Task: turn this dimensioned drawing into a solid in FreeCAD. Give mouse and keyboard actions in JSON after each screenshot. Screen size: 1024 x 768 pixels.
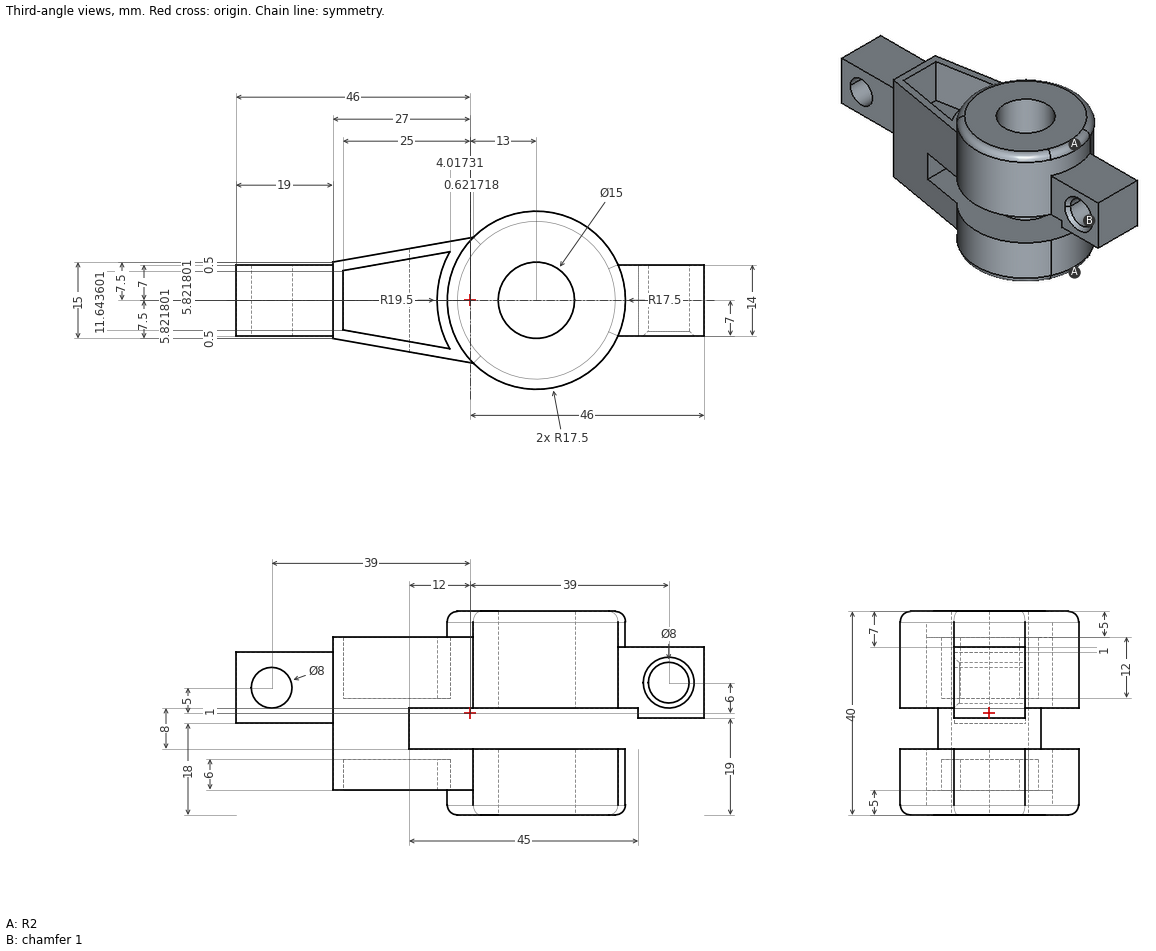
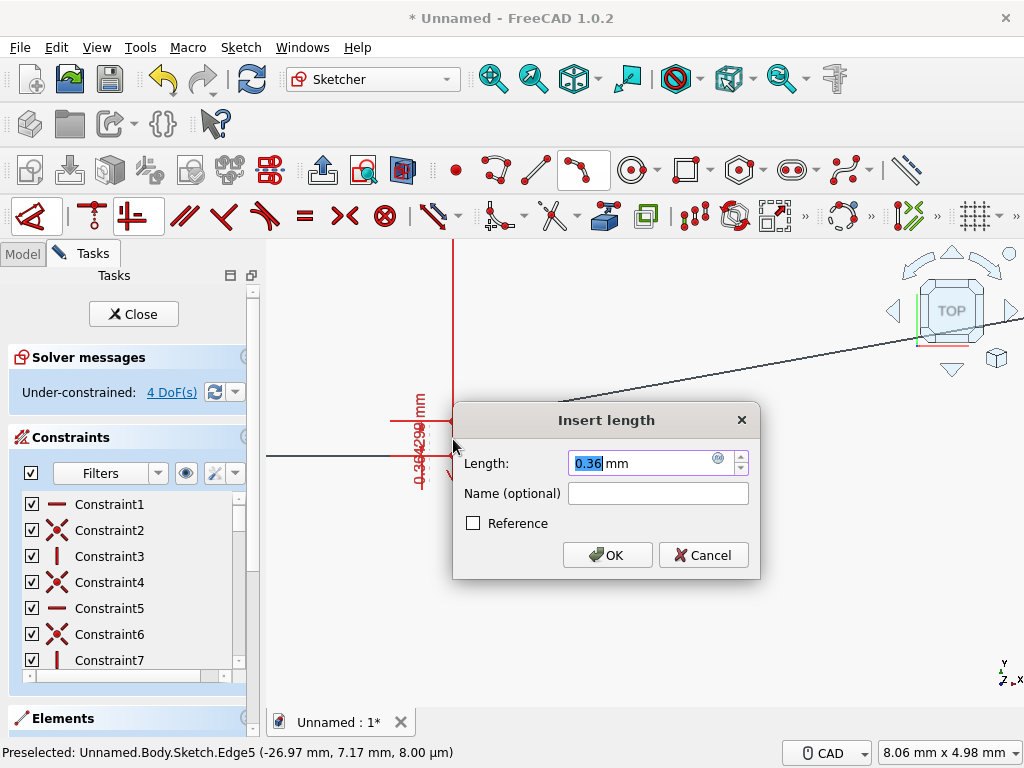
{"action": "type", "text": "0.5"}
{"action": "key", "text": "Return"}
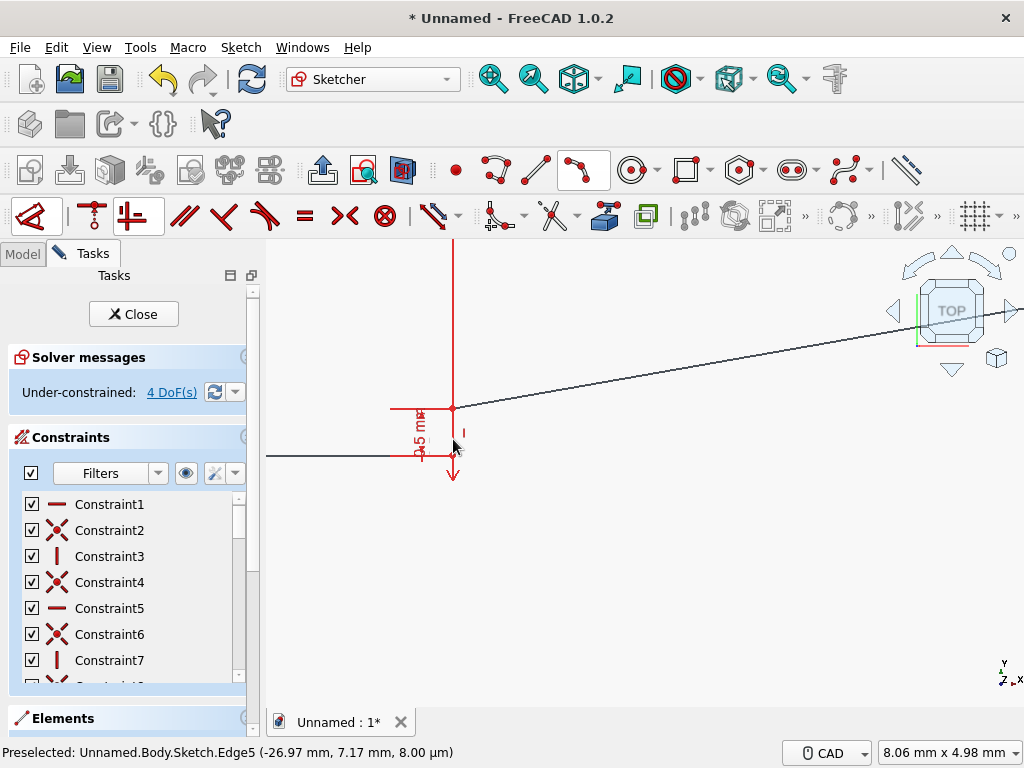
{"action": "scroll", "coordinate": [450, 439], "scroll_direction": "down", "scroll_amount": 15}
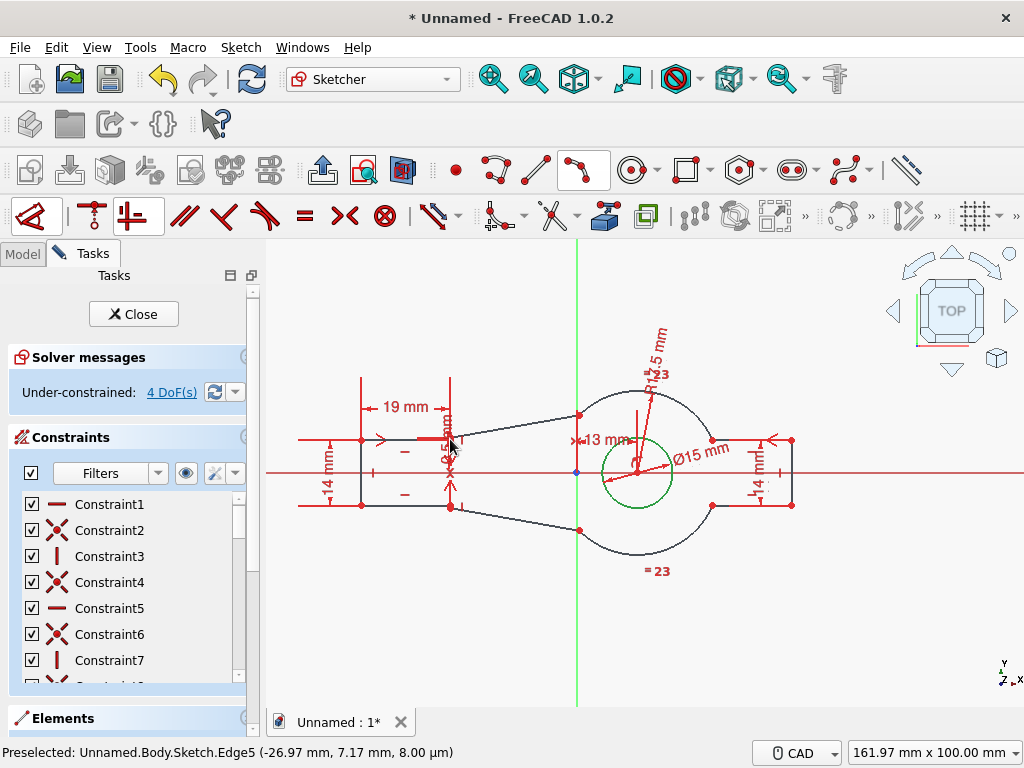
{"action": "scroll", "coordinate": [450, 506], "scroll_direction": "up", "scroll_amount": 15}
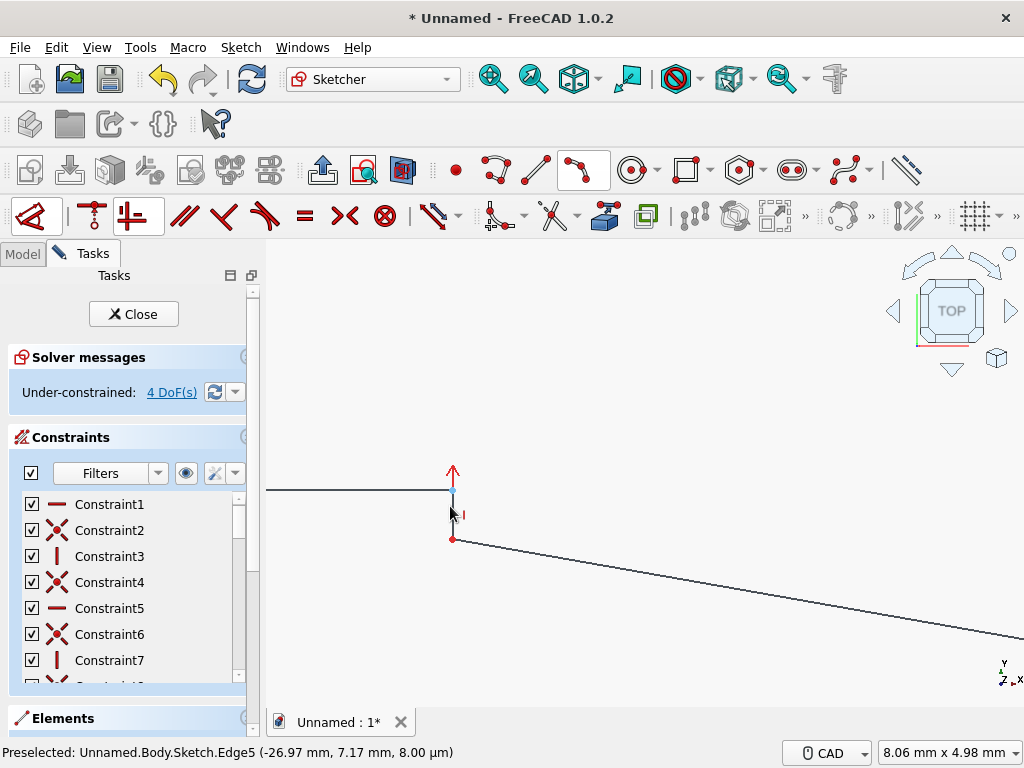
{"action": "left_click", "coordinate": [453, 505]}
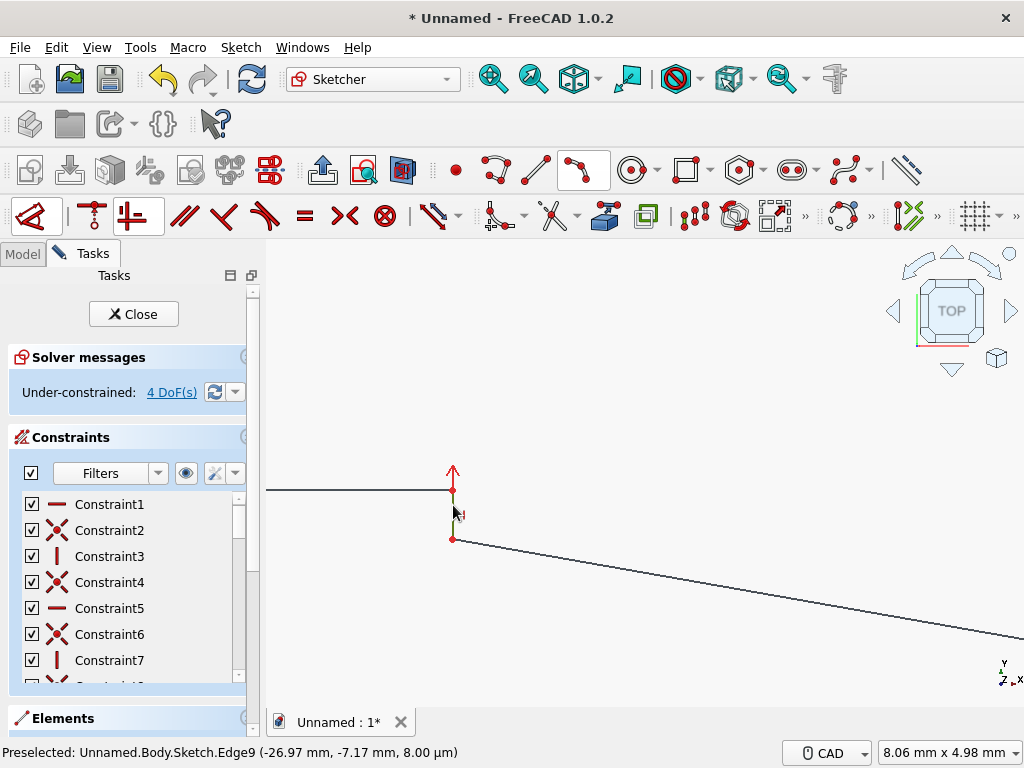
{"action": "key", "text": "i"}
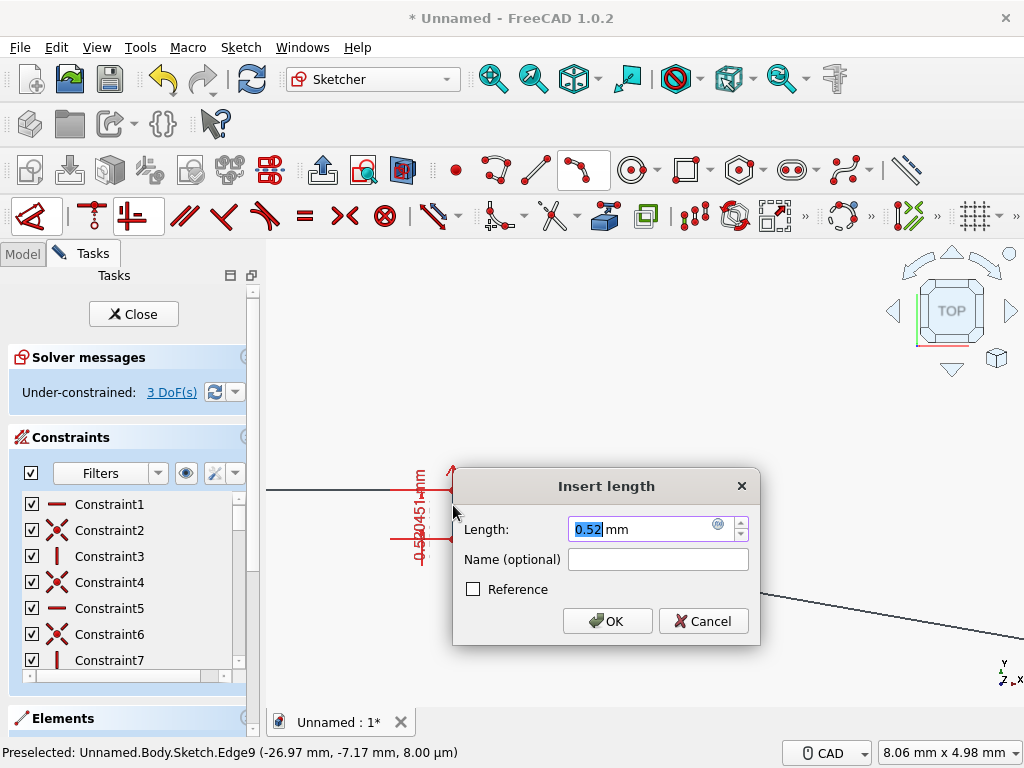
{"action": "type", "text": "0.5"}
{"action": "key", "text": "Return"}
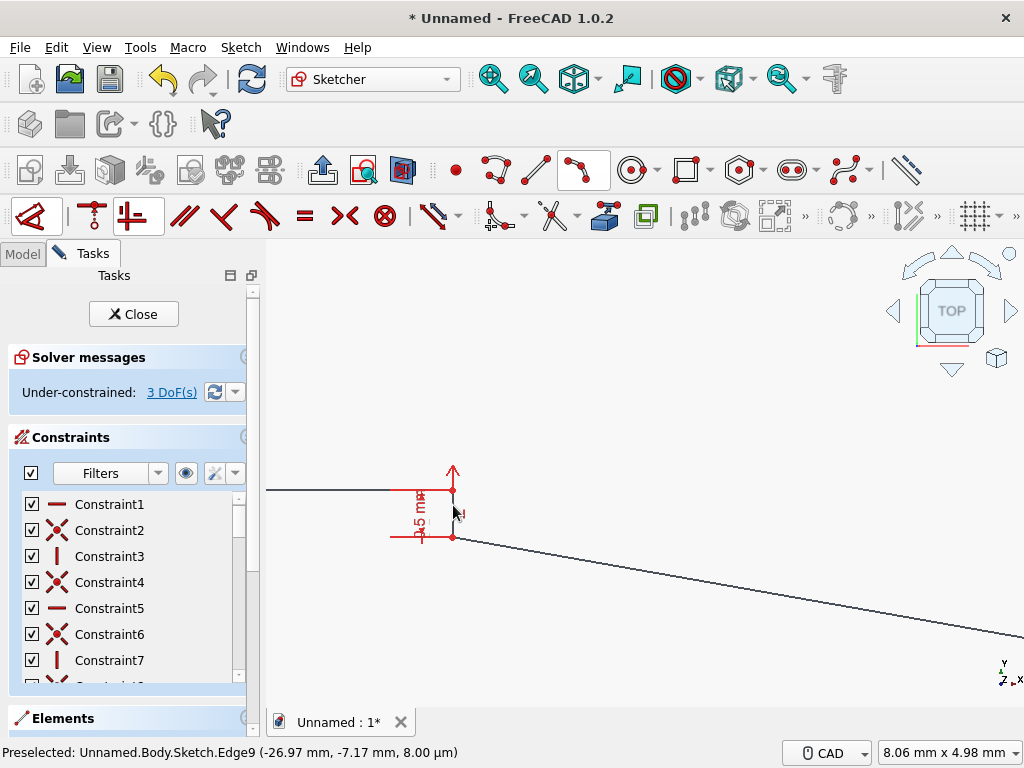
{"action": "scroll", "coordinate": [450, 507], "scroll_direction": "down", "scroll_amount": 15}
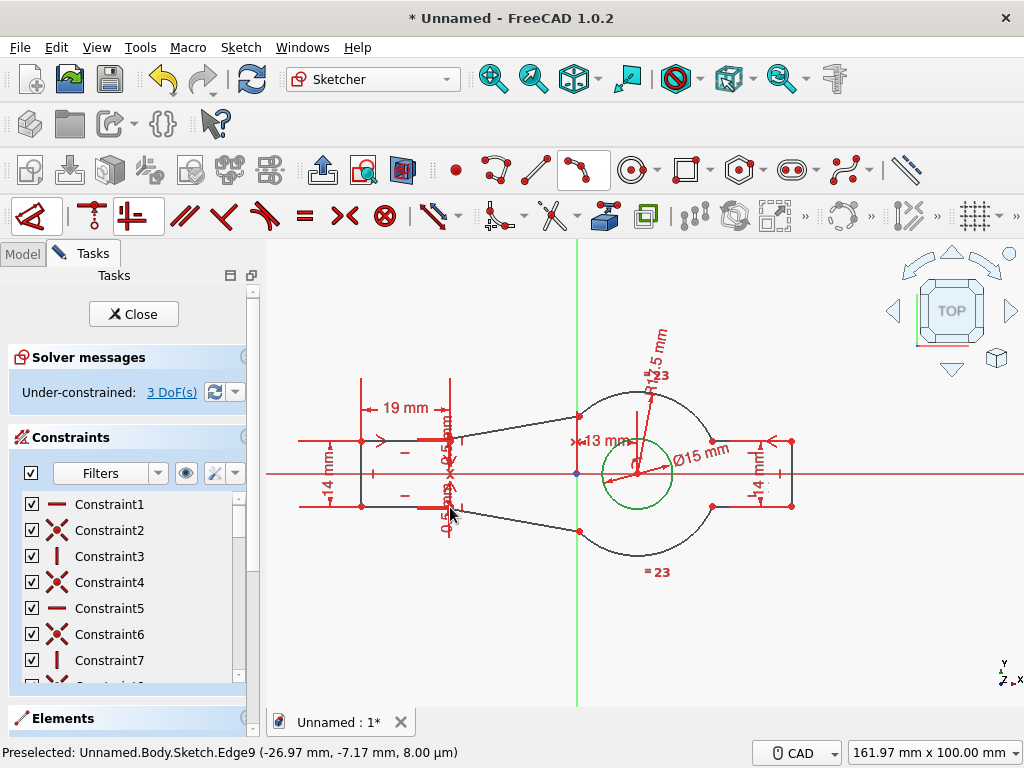
{"action": "left_click", "coordinate": [792, 507]}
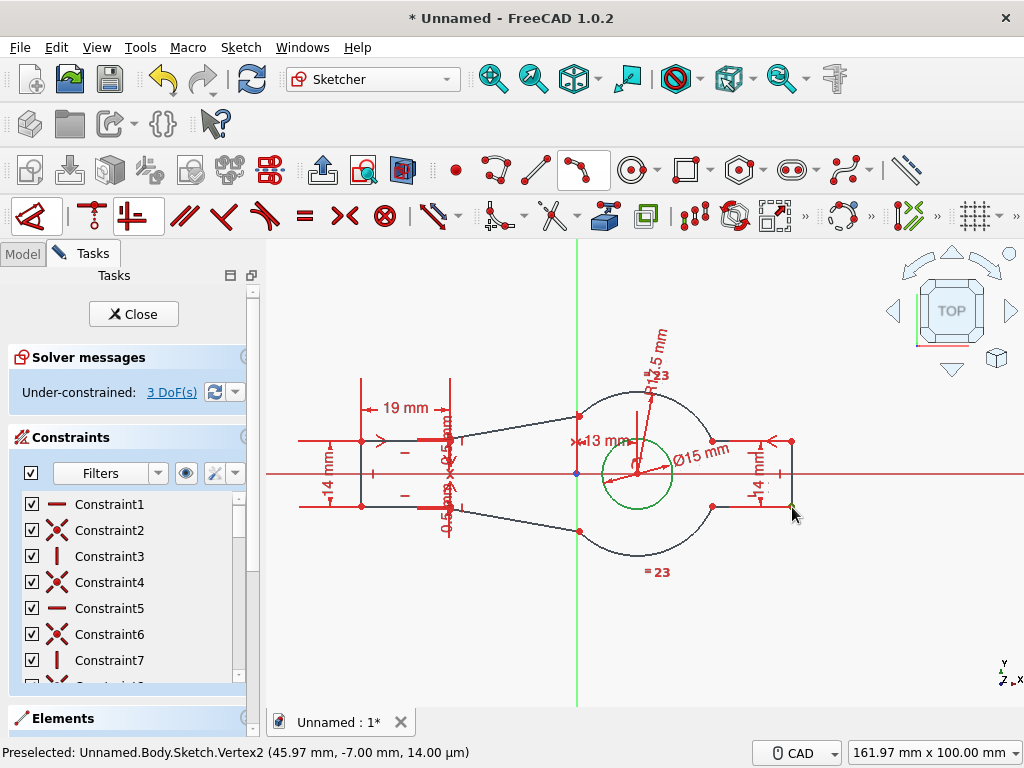
{"action": "left_click", "coordinate": [56, 216]}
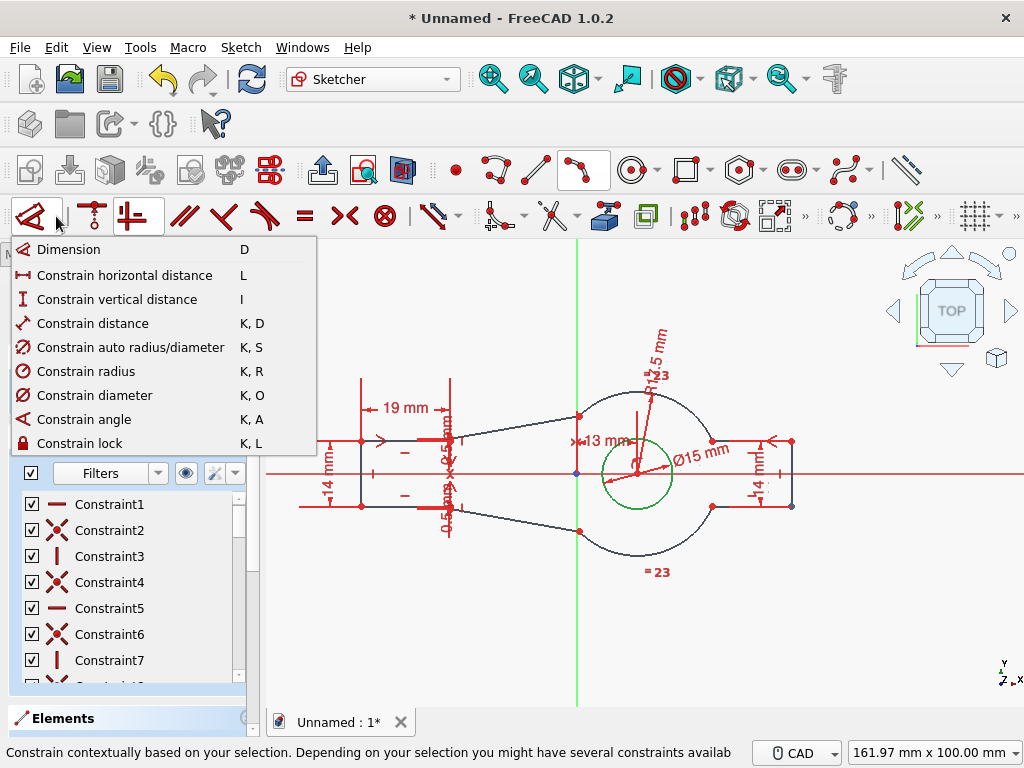
{"action": "left_click", "coordinate": [164, 275]}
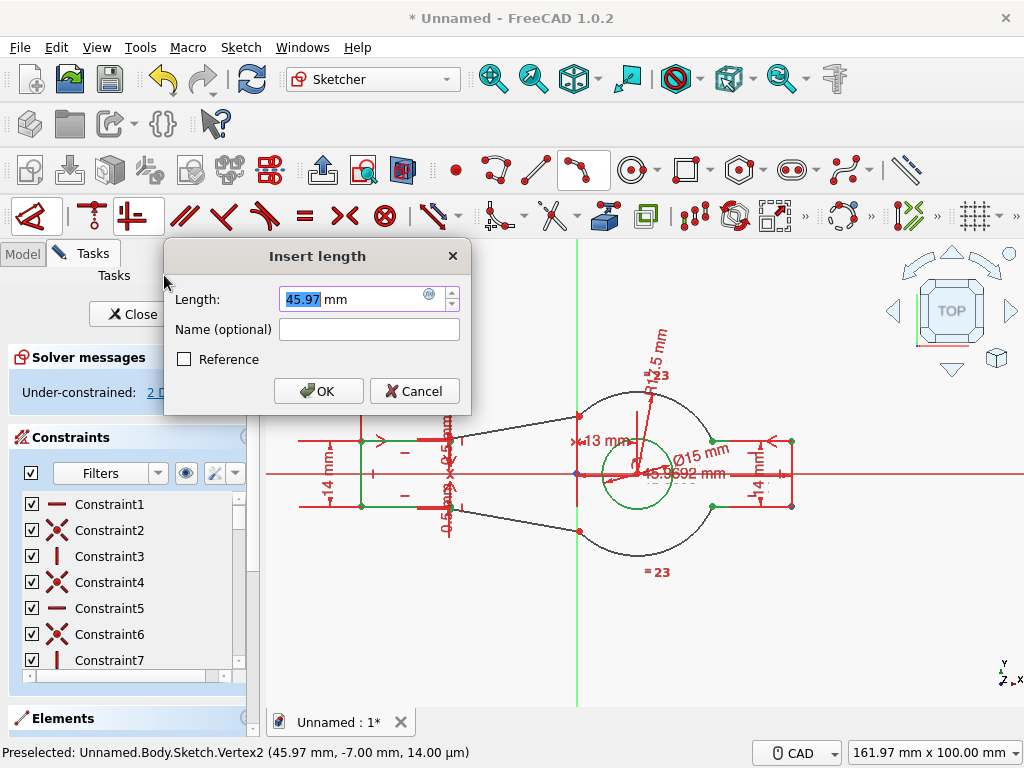
{"action": "type", "text": "46"}
{"action": "key", "text": "Return"}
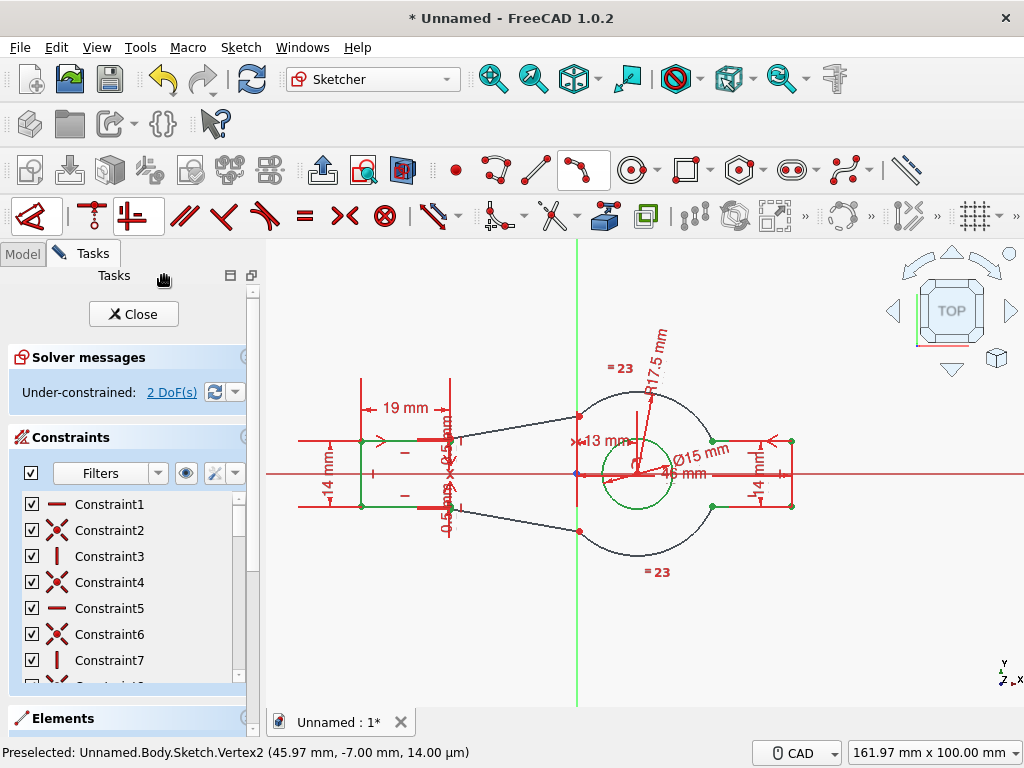
{"action": "scroll", "coordinate": [579, 416], "scroll_direction": "up", "scroll_amount": 14}